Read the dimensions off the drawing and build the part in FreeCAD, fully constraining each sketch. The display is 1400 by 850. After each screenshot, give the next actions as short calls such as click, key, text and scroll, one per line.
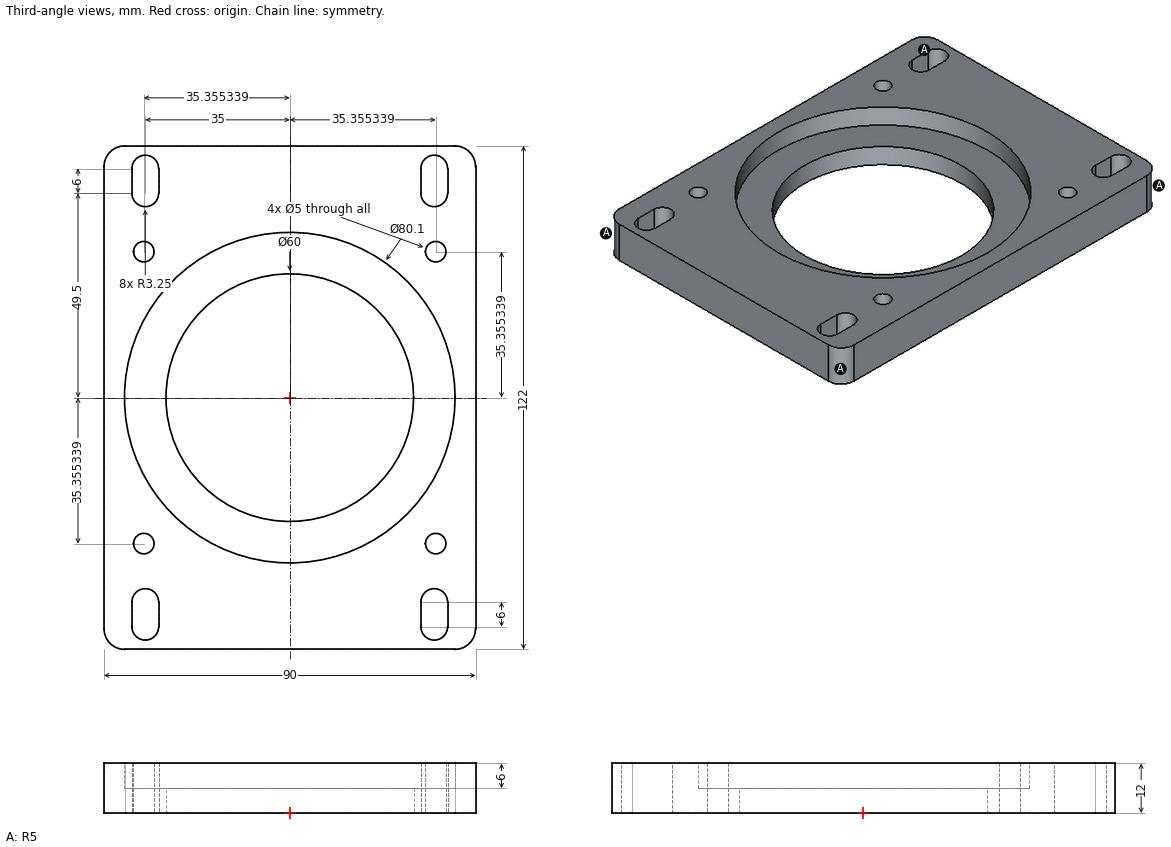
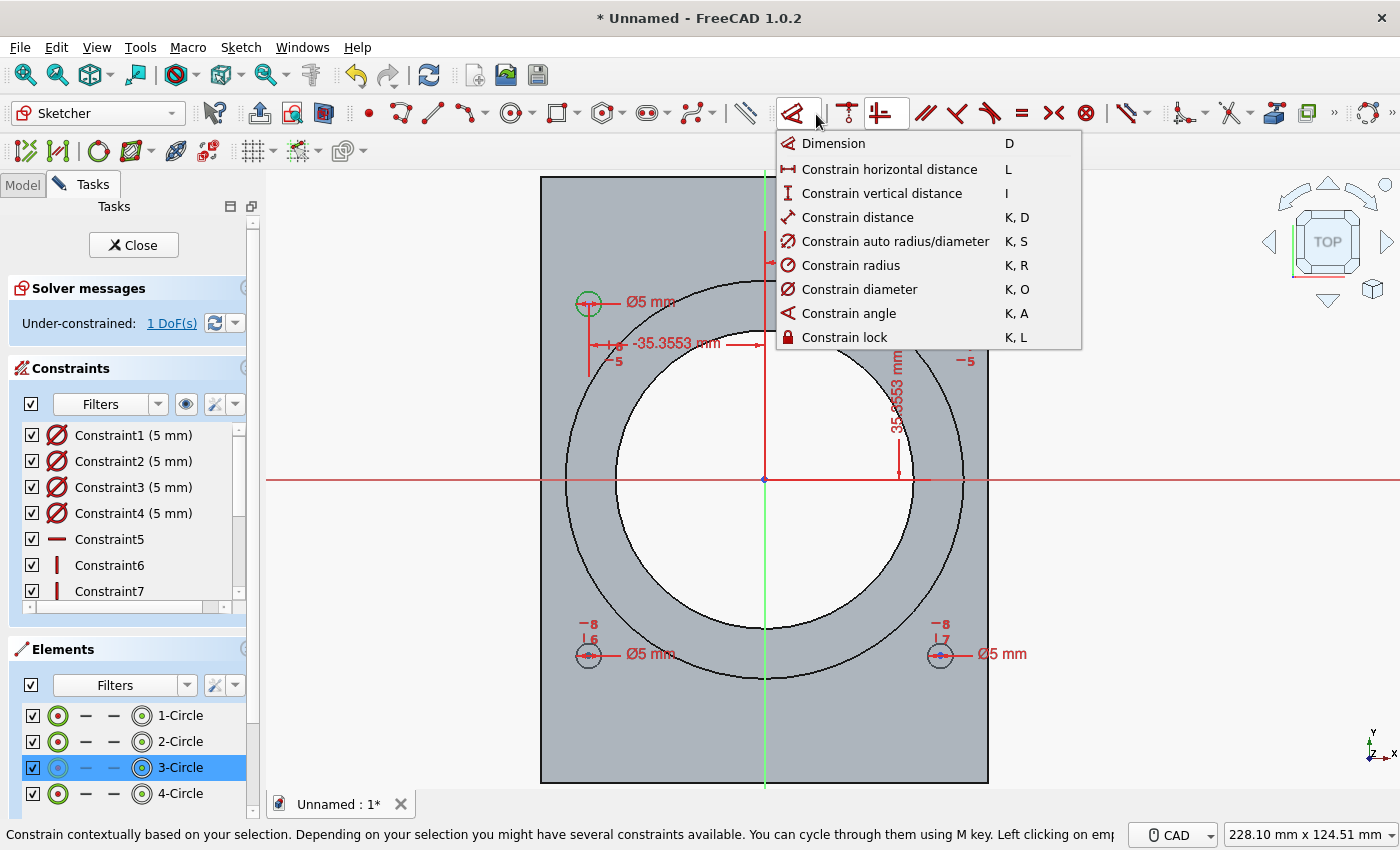
click(929, 193)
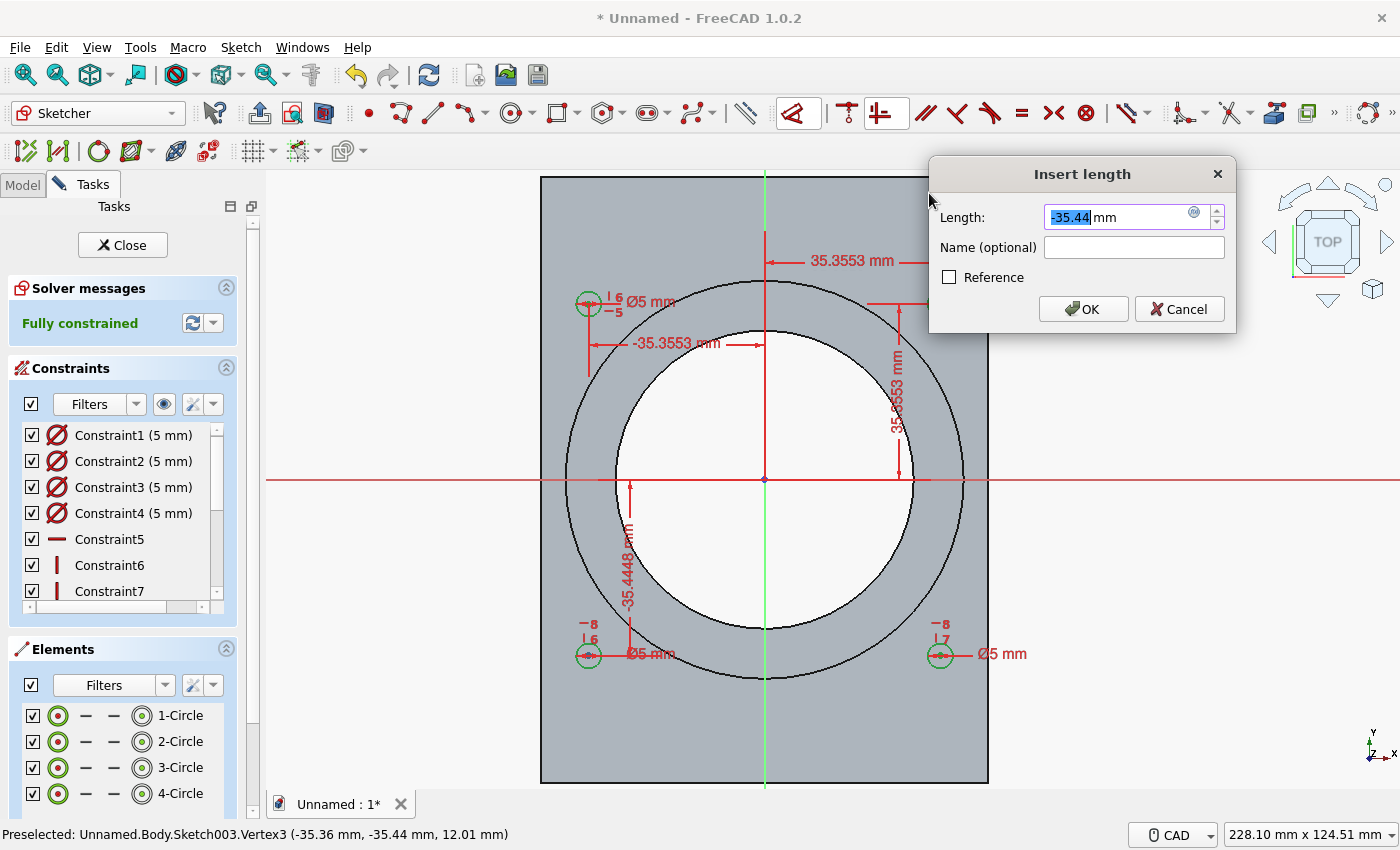
text(-35.355339)
key(Return)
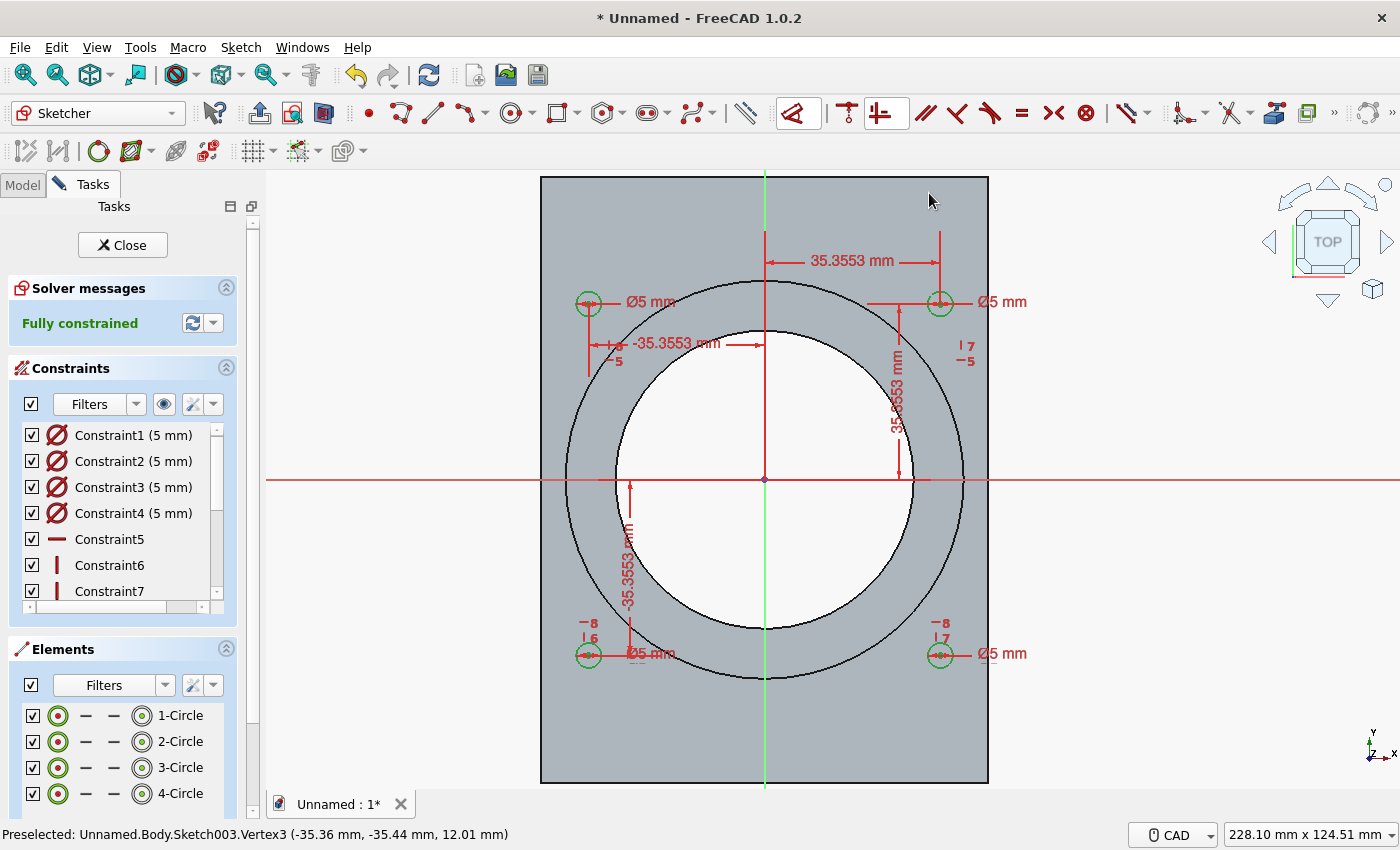
click(123, 245)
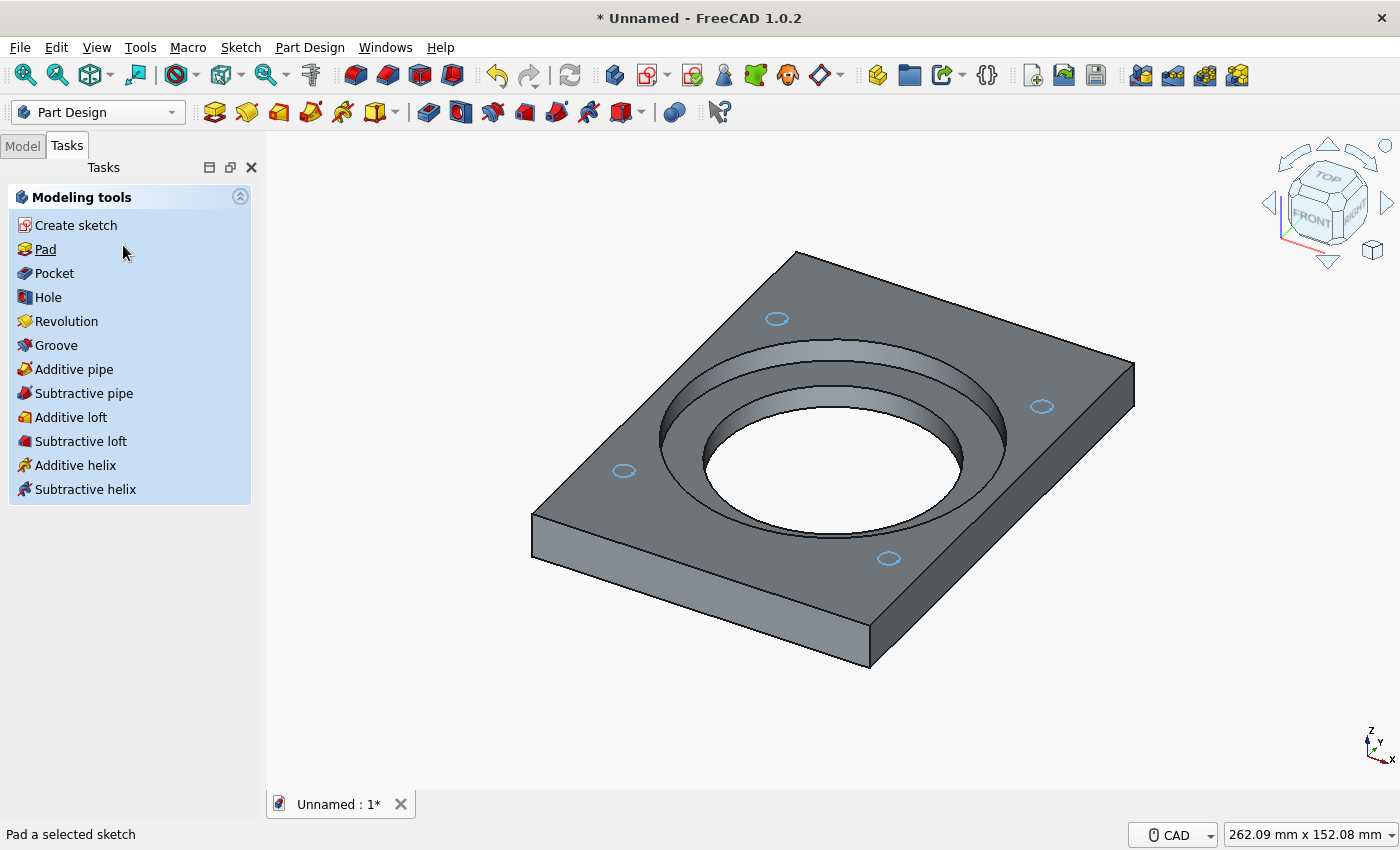
click(462, 112)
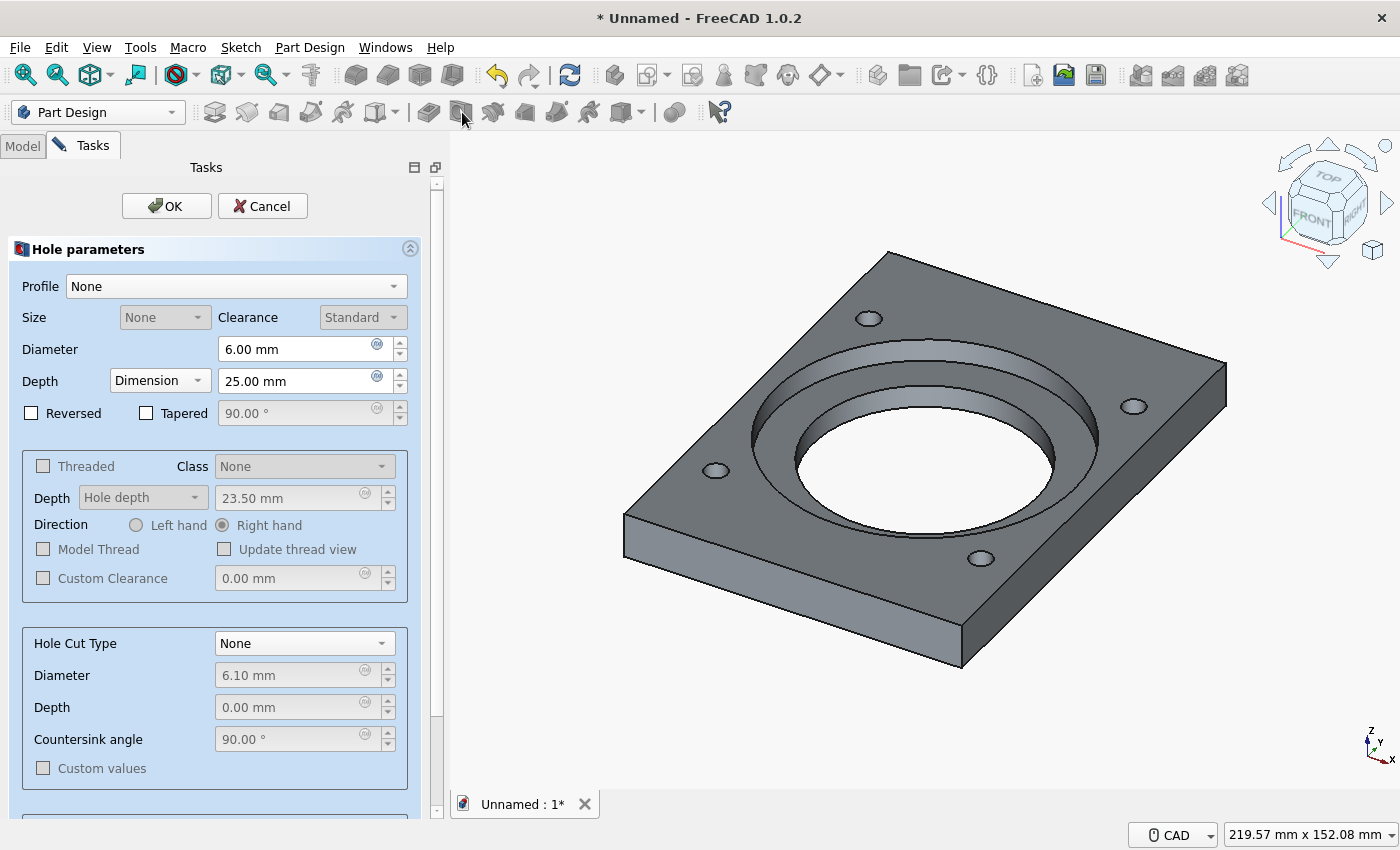
triple_click(305, 349)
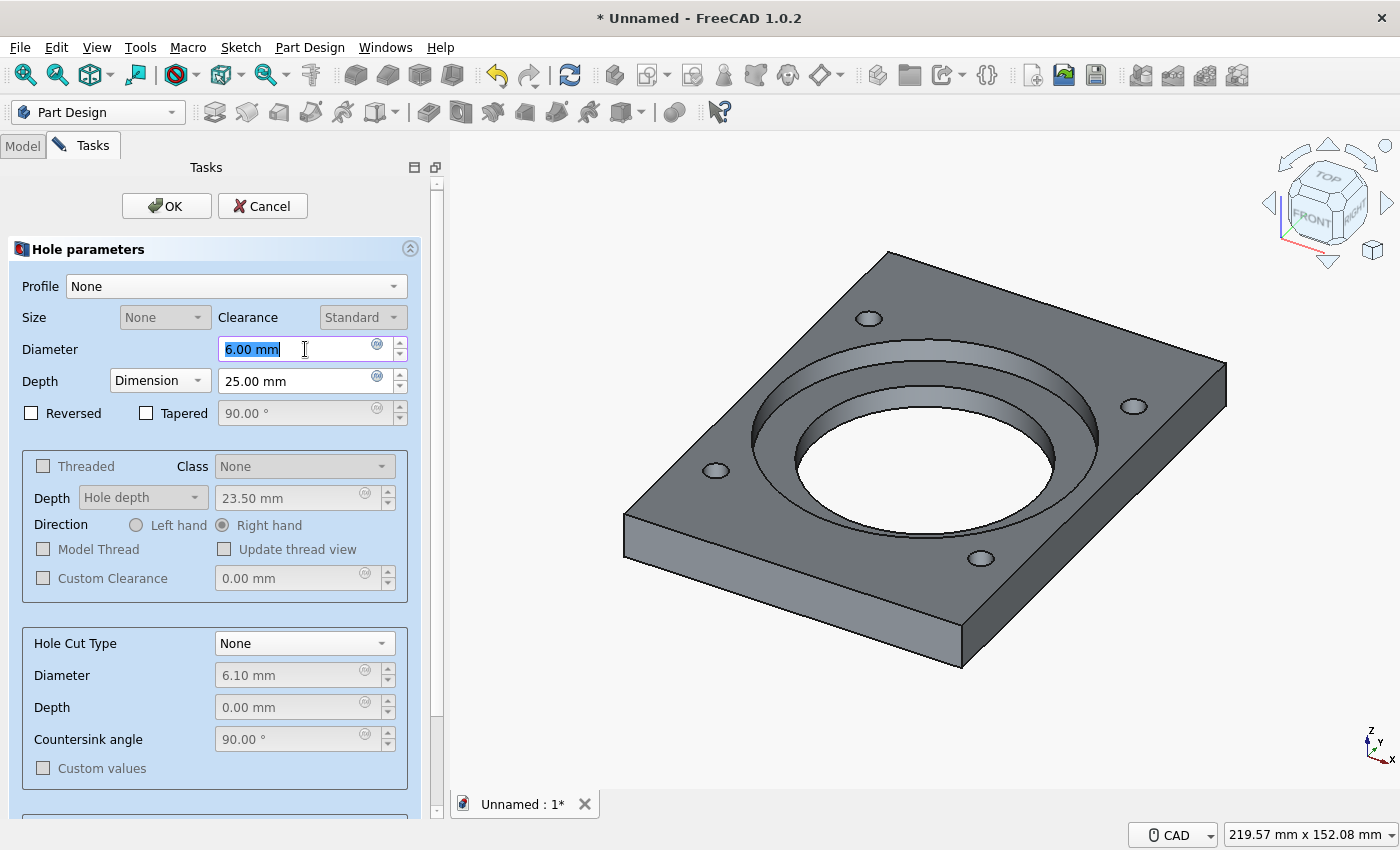
text(5)
key(Tab)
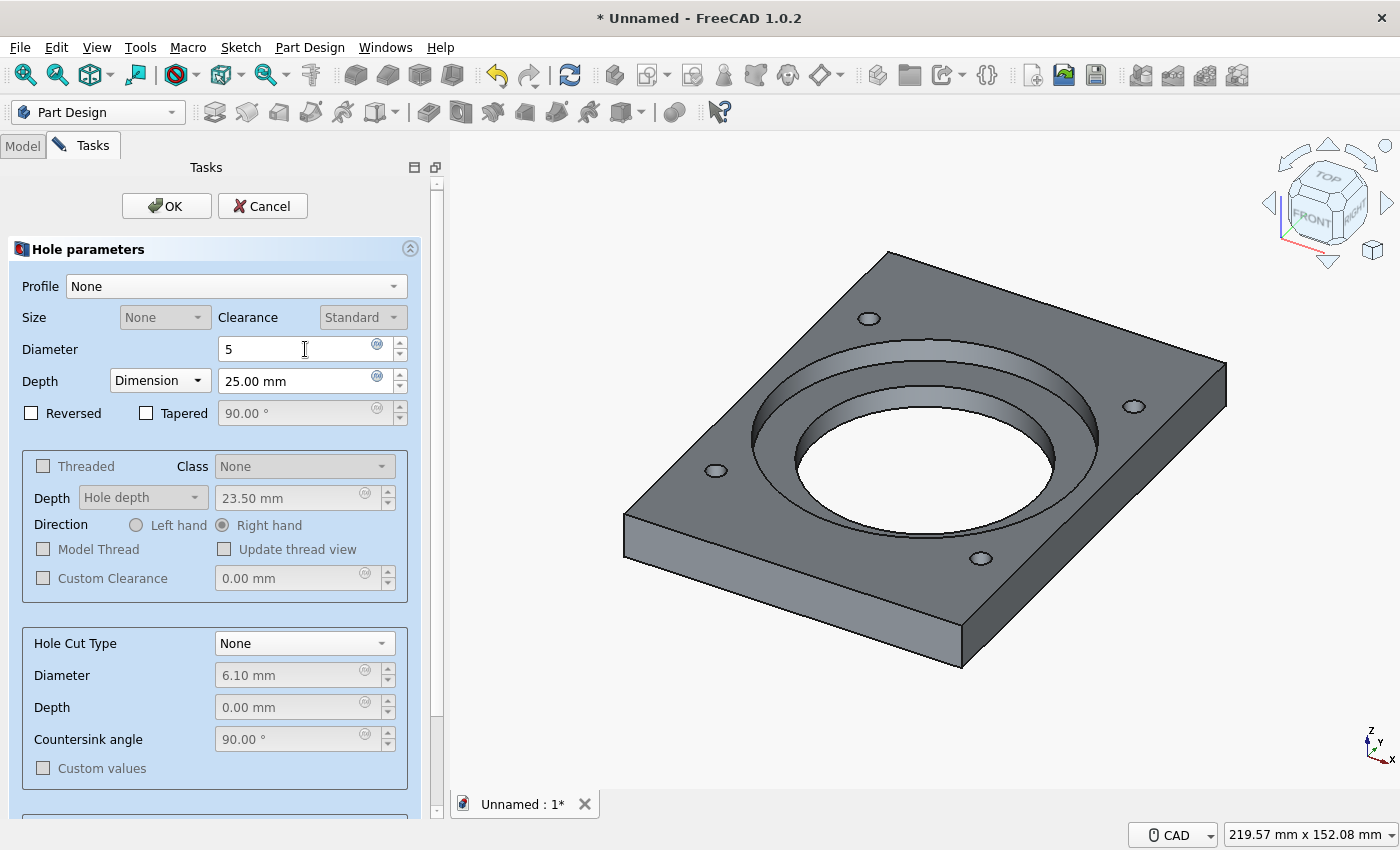
click(161, 380)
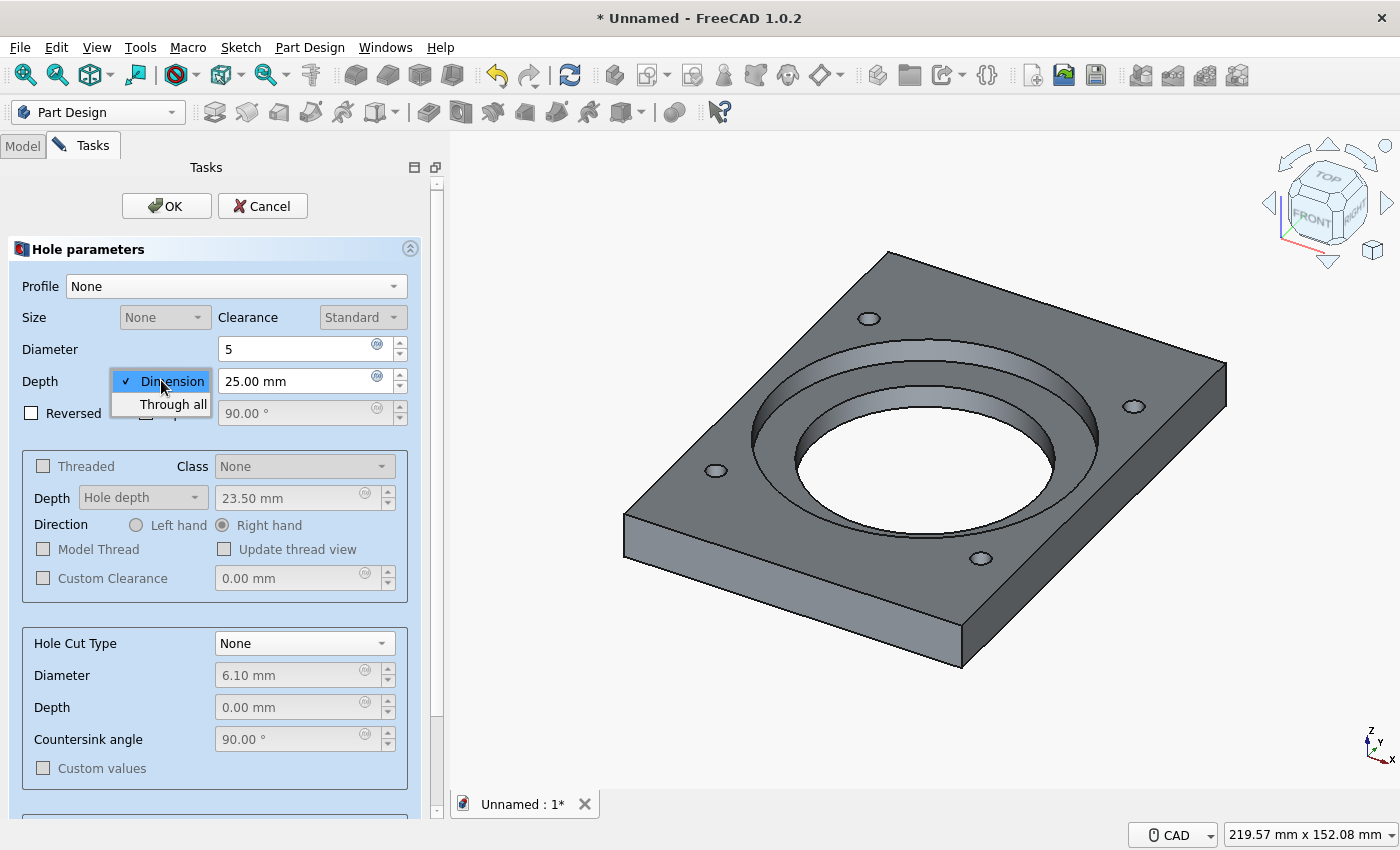
click(160, 404)